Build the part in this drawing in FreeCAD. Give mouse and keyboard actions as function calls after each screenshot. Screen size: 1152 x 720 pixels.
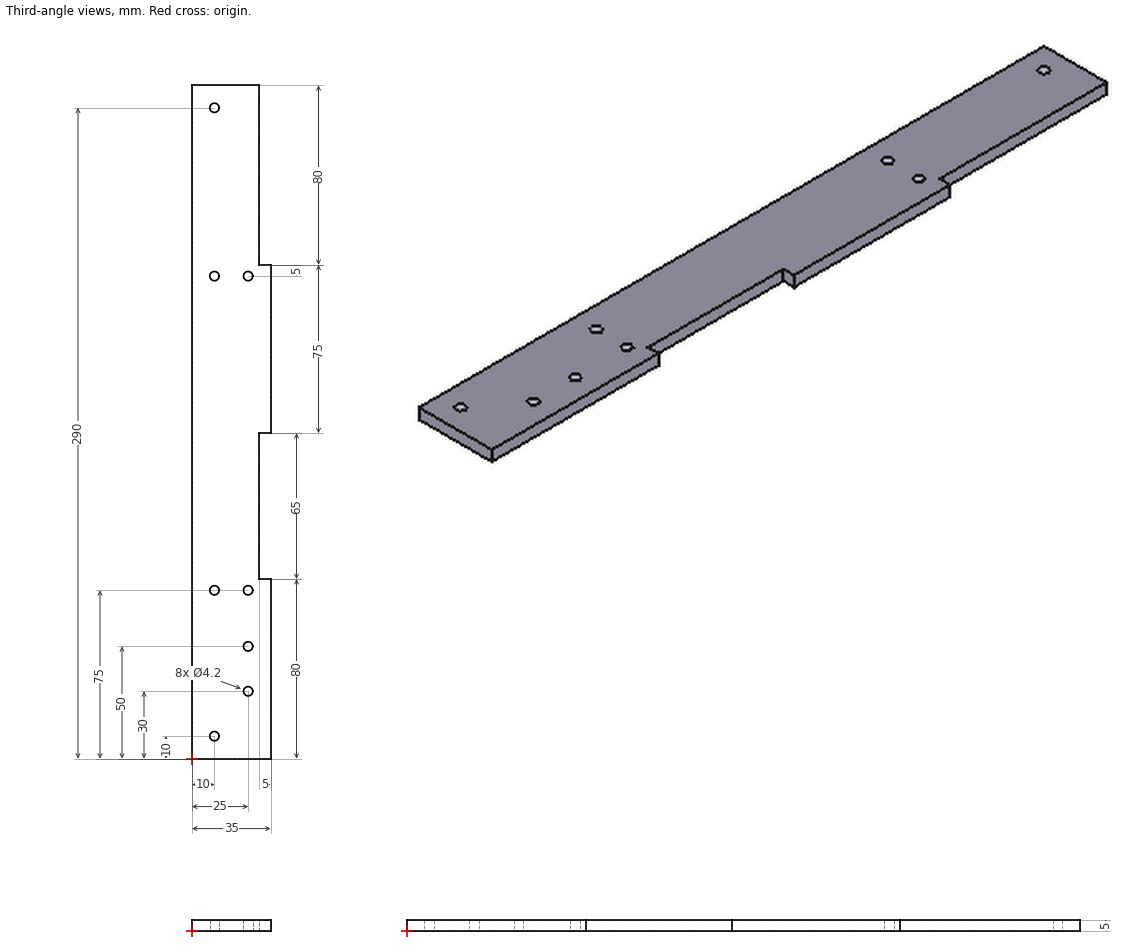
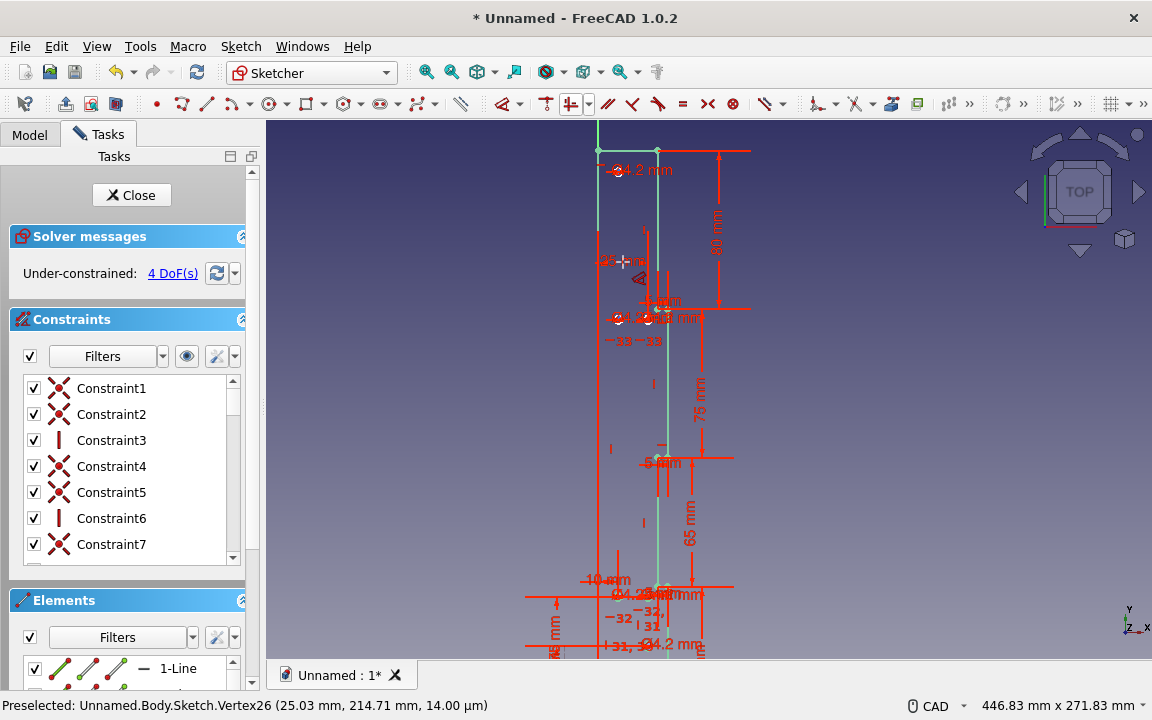
scroll(618, 320, up, 4)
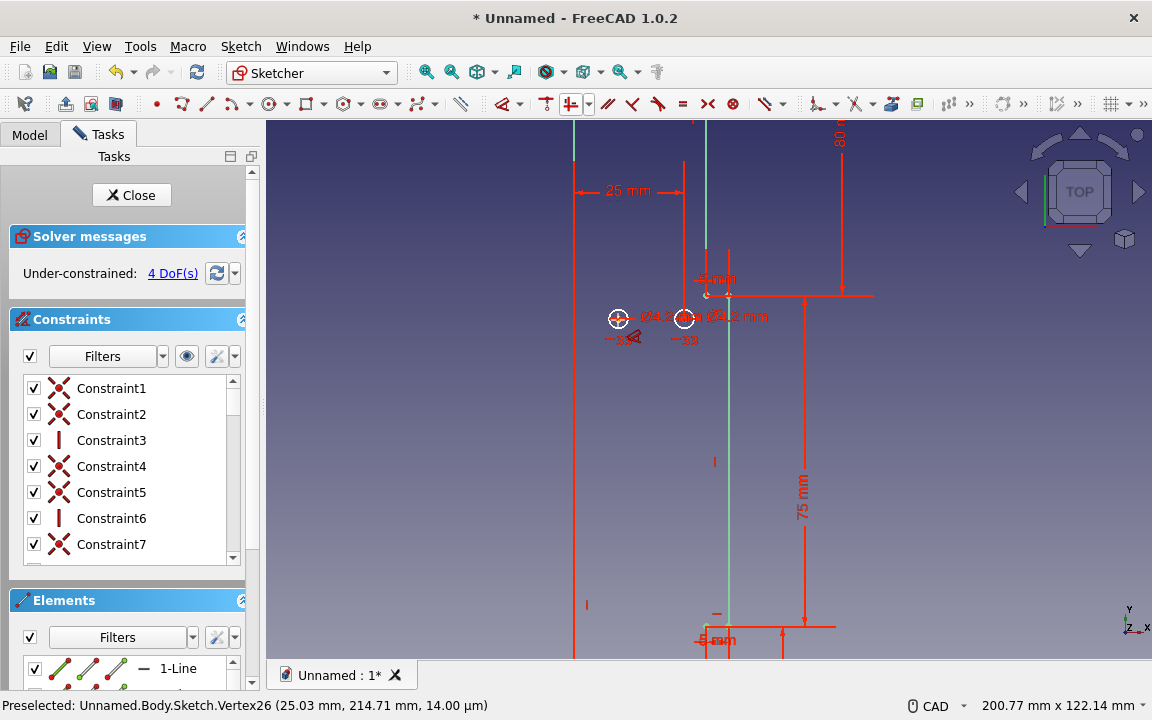
click(619, 319)
click(596, 285)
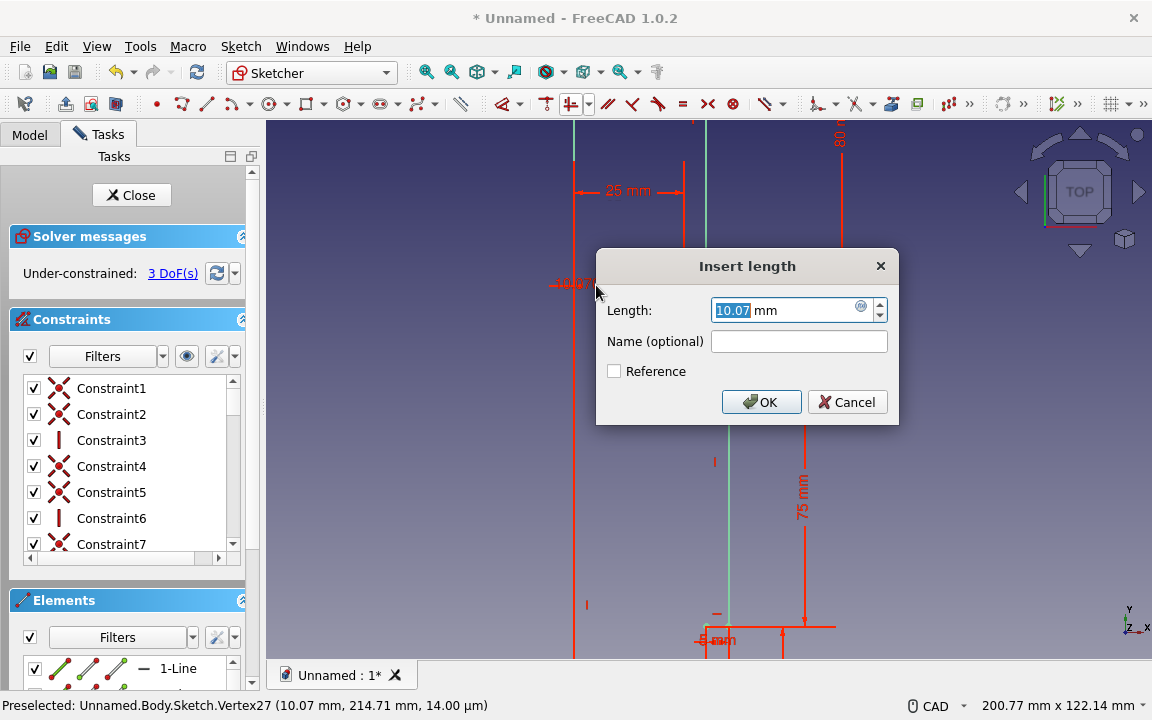
text(10)
key(Return)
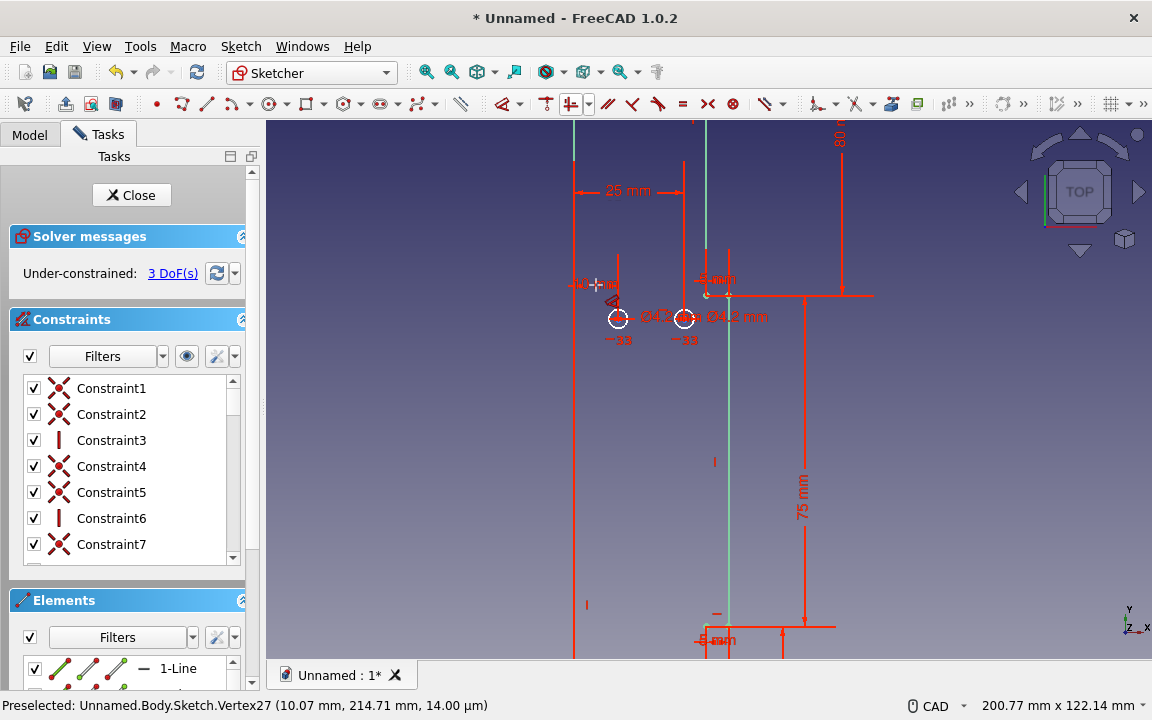
scroll(637, 319, down, 7)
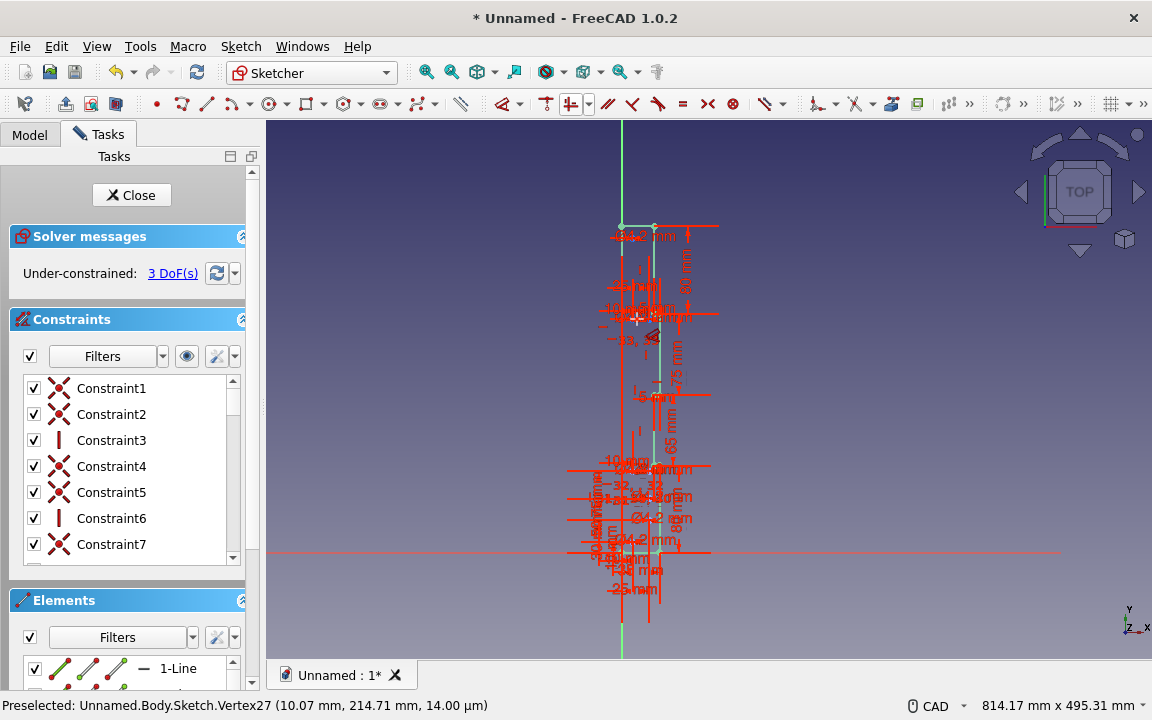
scroll(633, 238, up, 7)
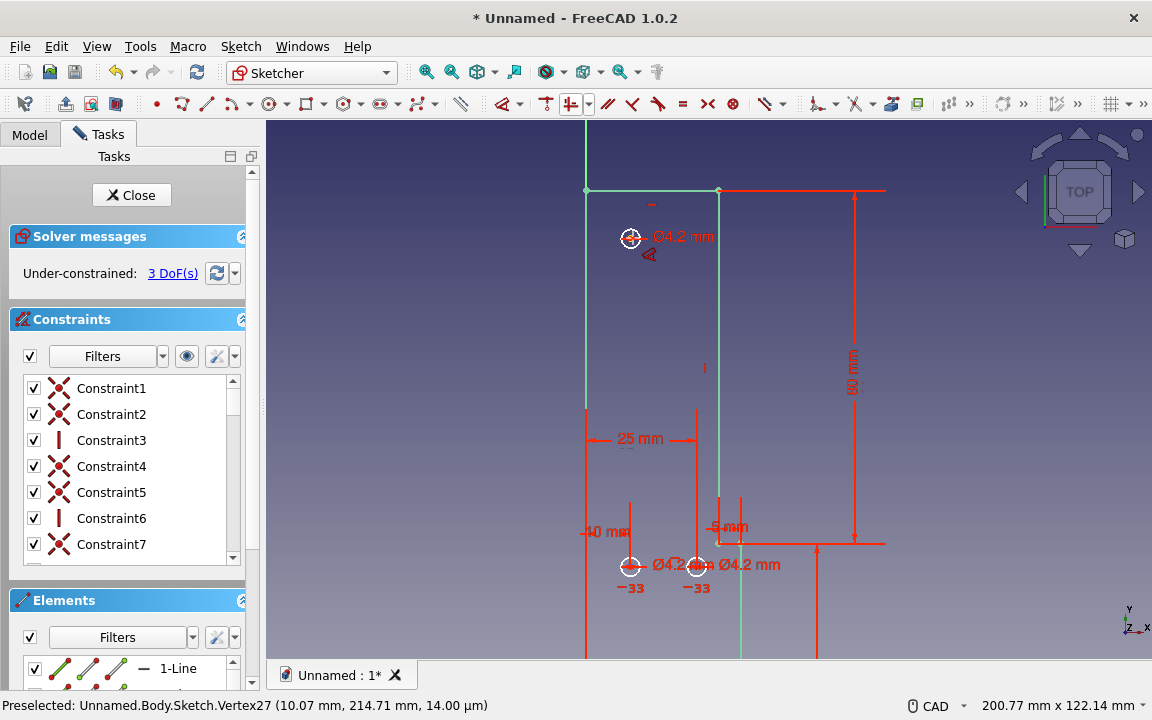
click(631, 239)
click(609, 205)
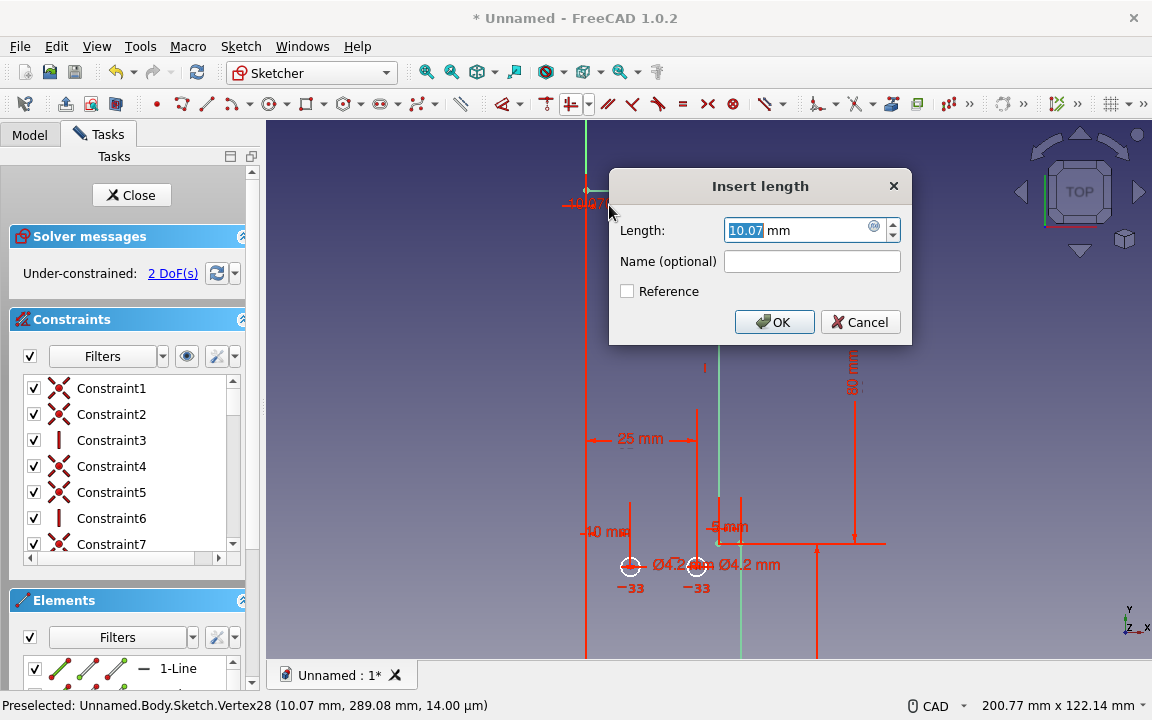
text(10)
key(Return)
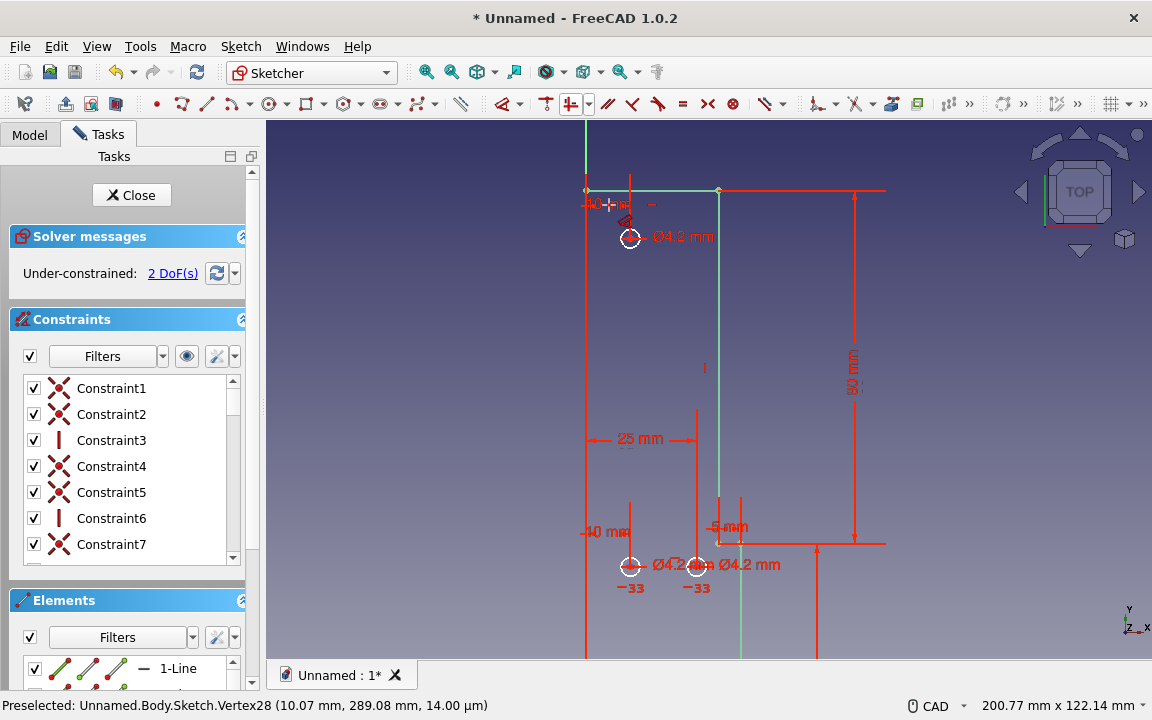
scroll(719, 544, up, 3)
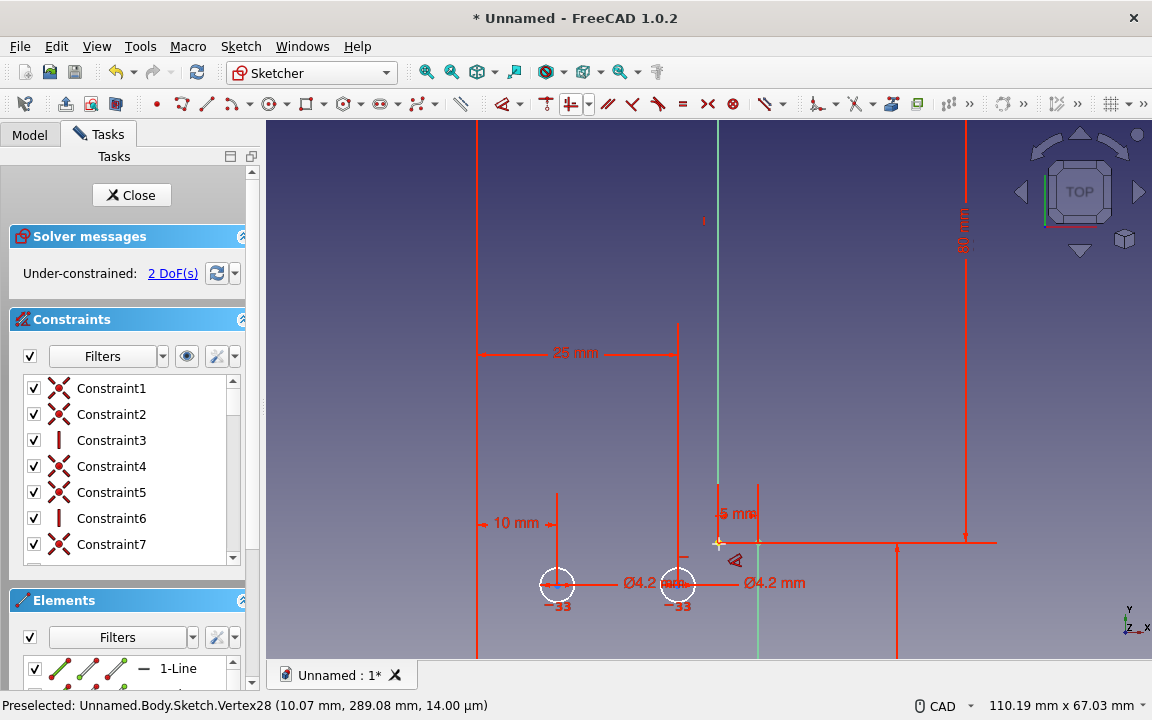
click(718, 543)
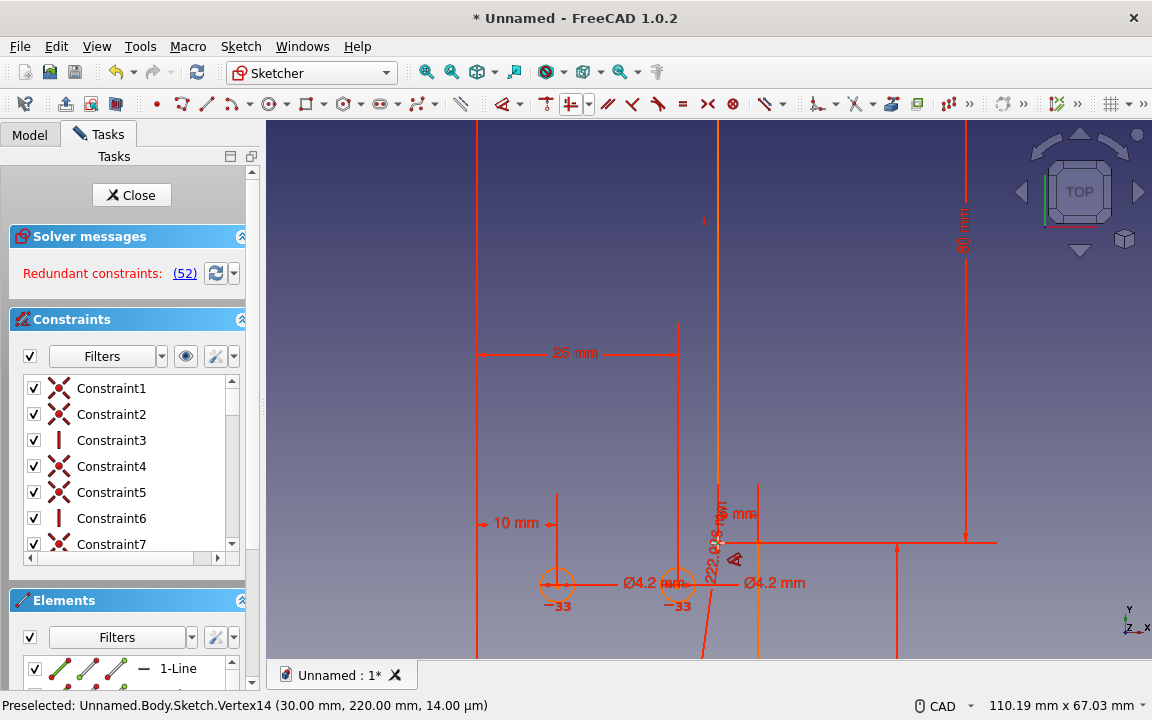
click(678, 585)
click(644, 564)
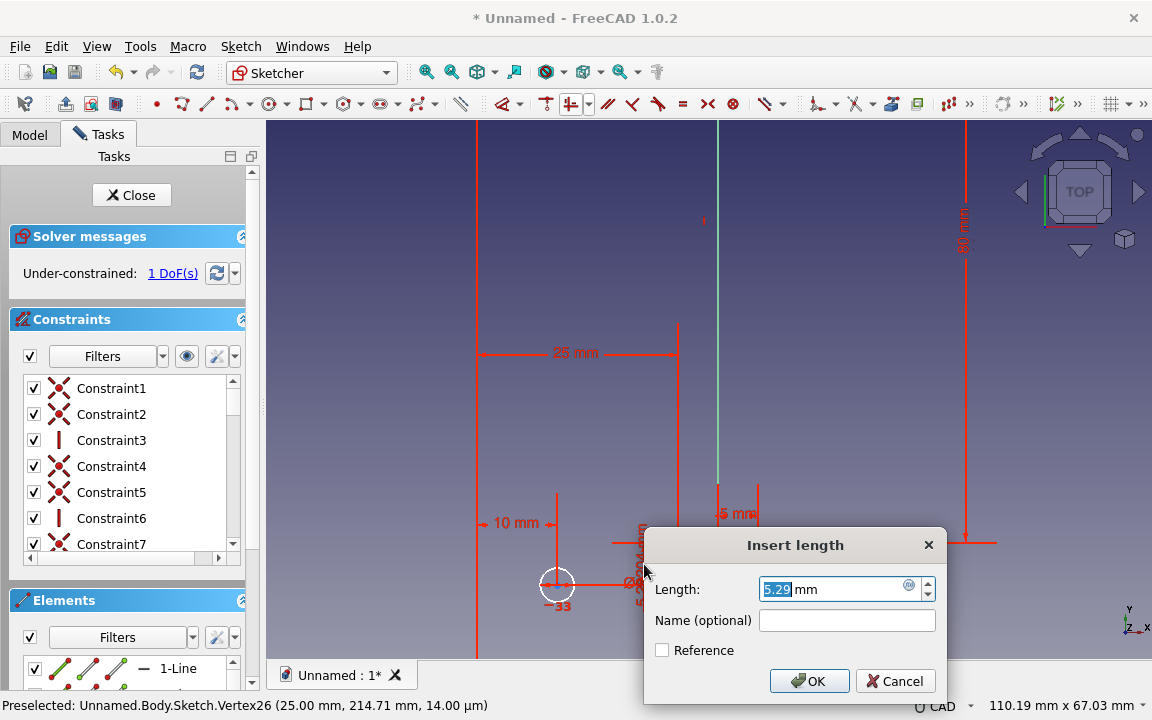
text(5)
key(Return)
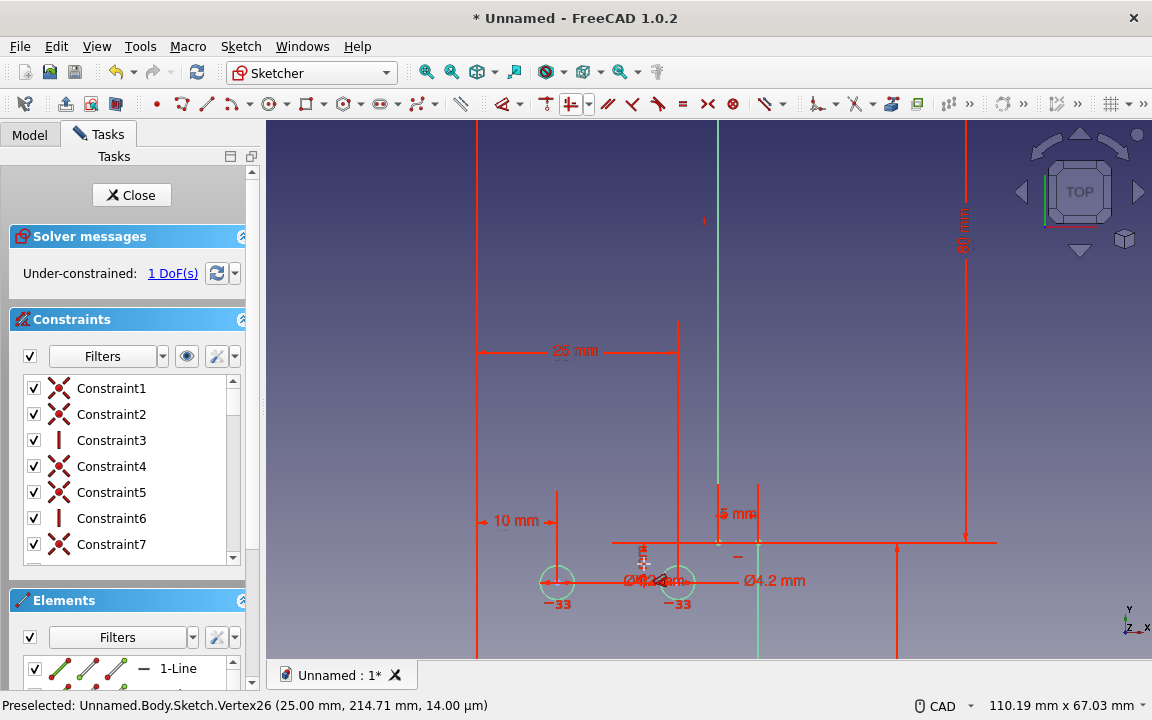
scroll(644, 277, down, 10)